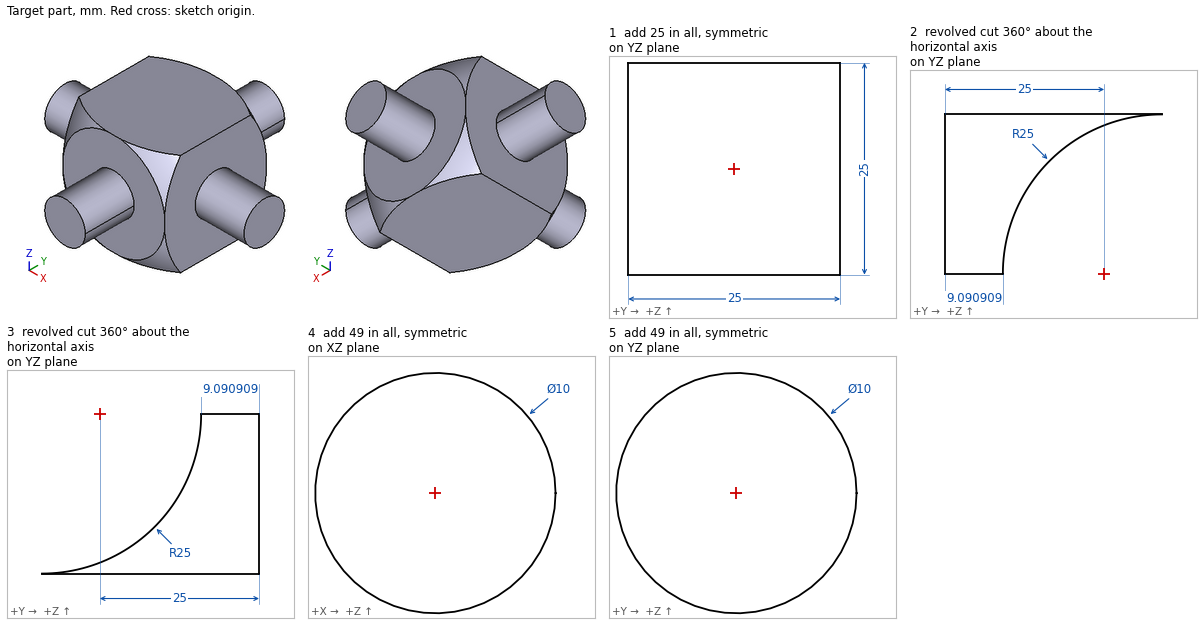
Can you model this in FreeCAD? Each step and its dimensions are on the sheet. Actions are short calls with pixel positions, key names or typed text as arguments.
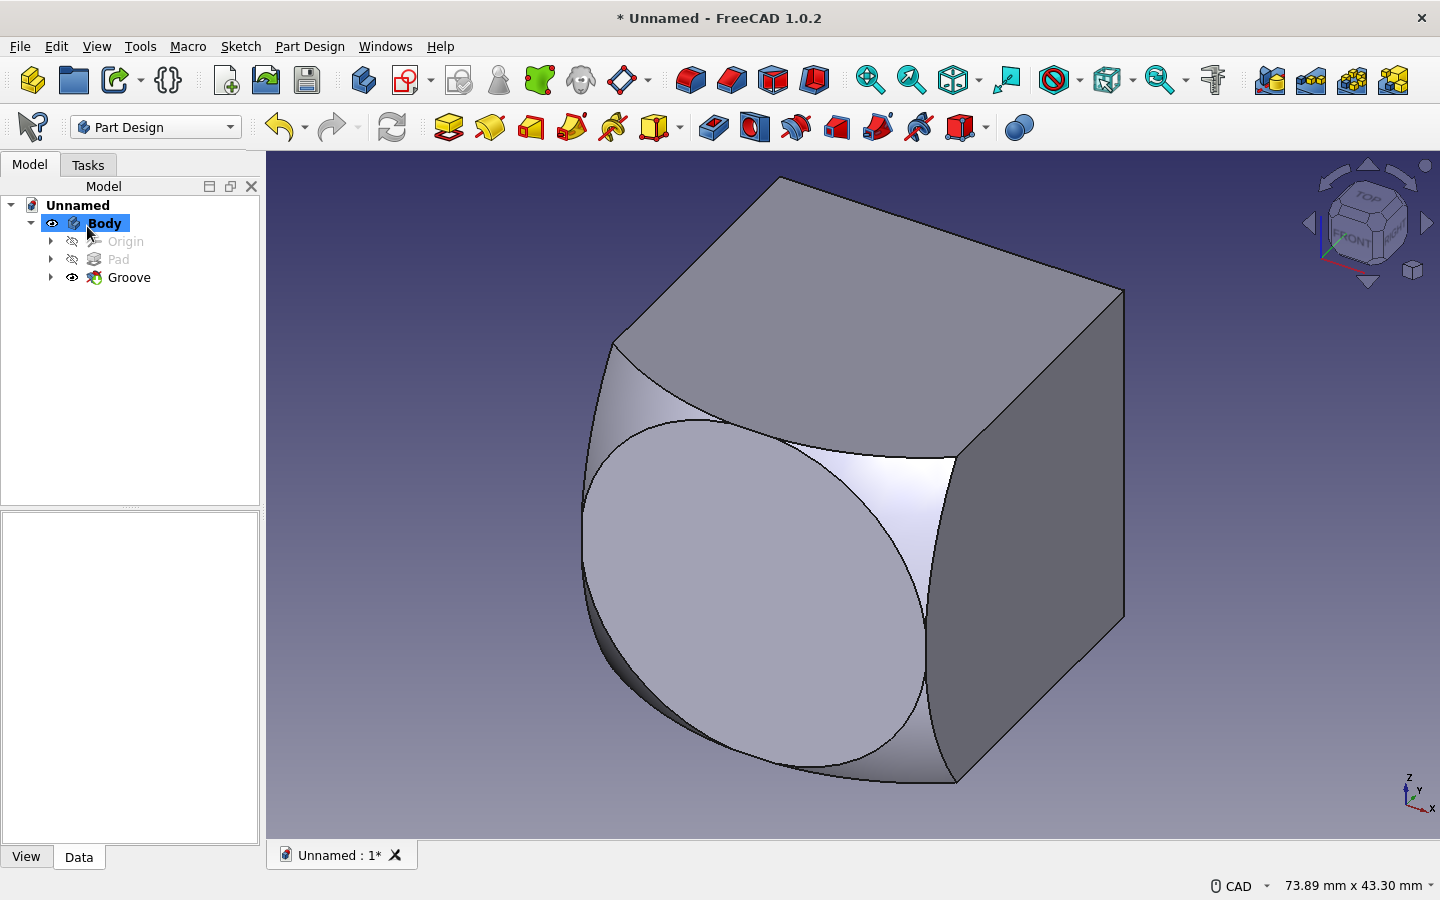
click(404, 80)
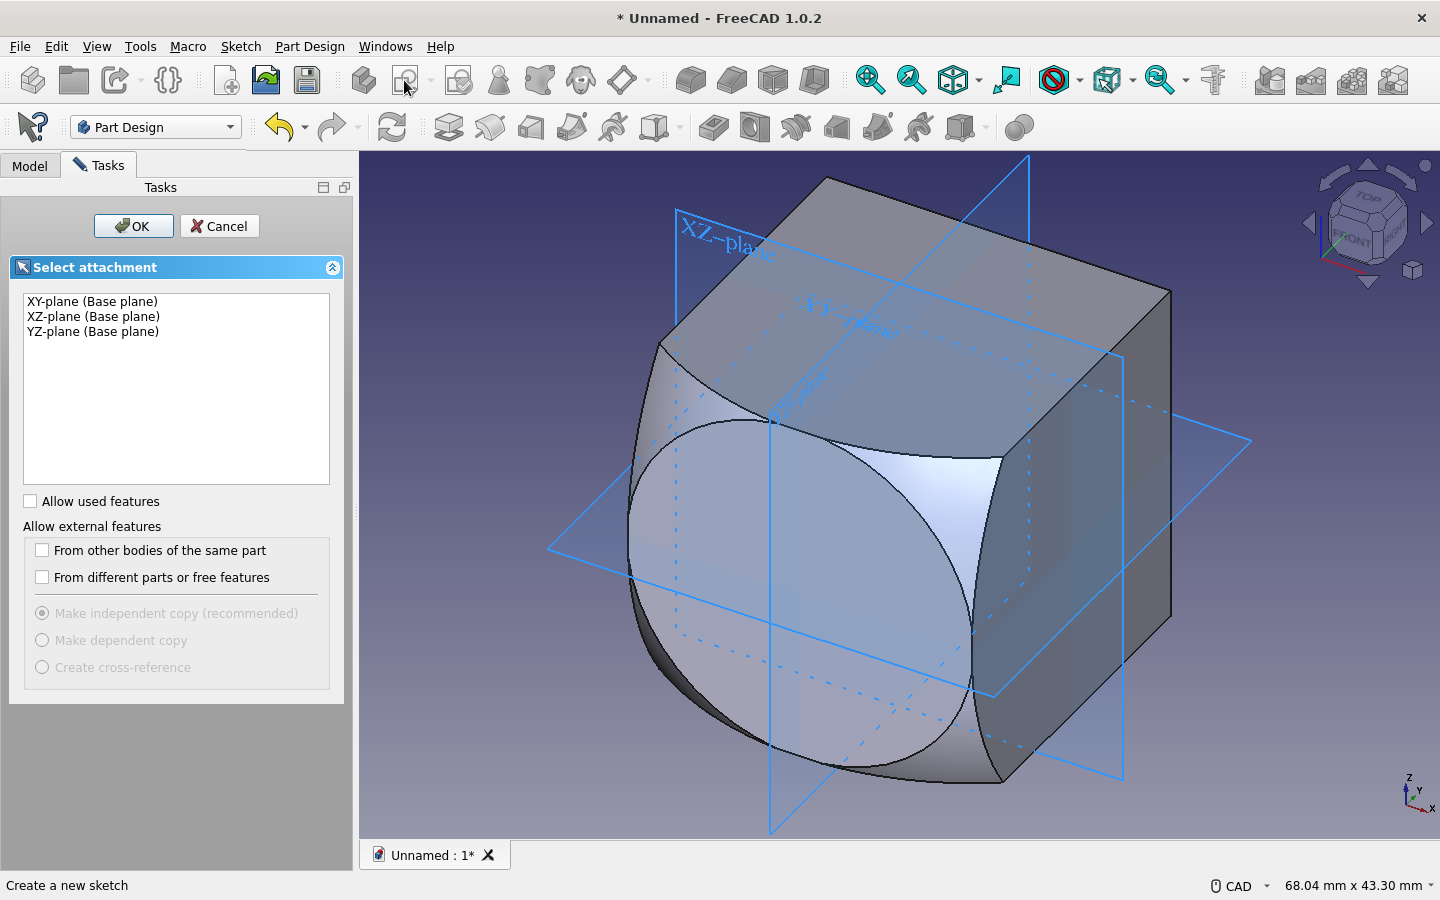
click(84, 332)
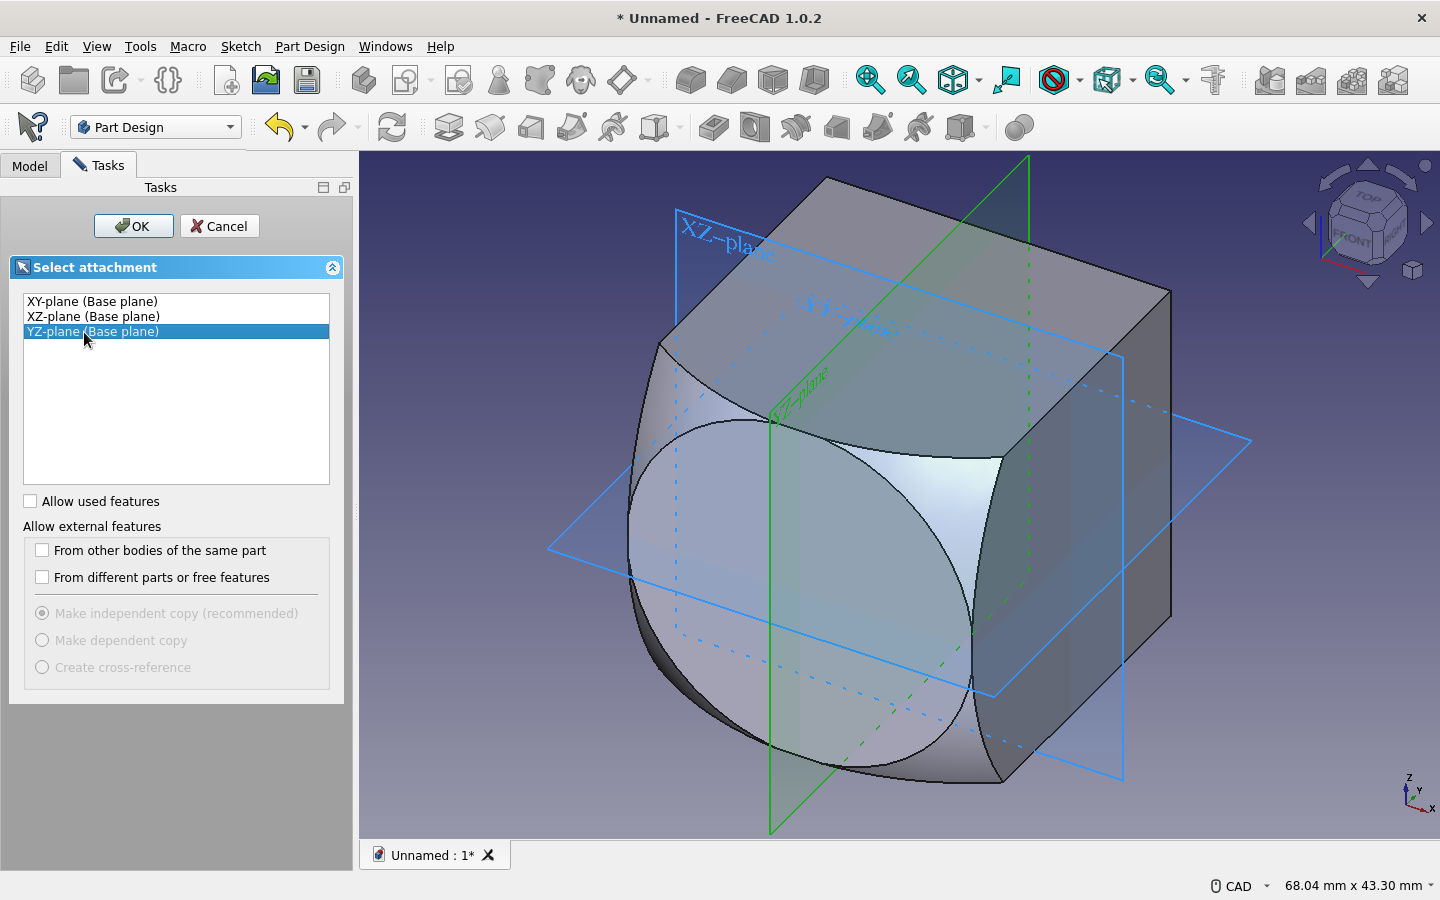
click(134, 226)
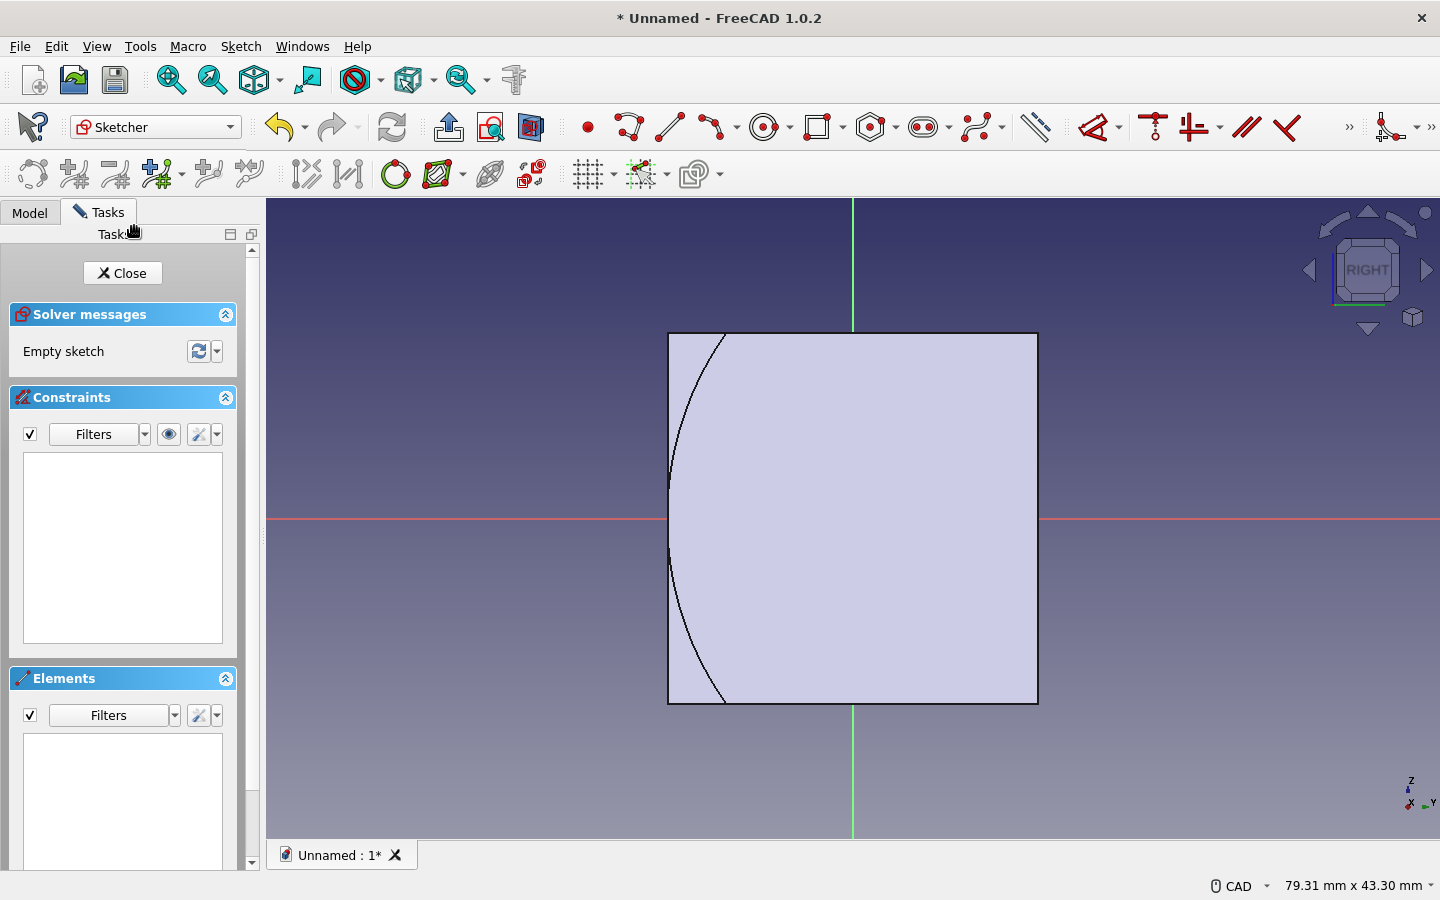
key(q)
key(s)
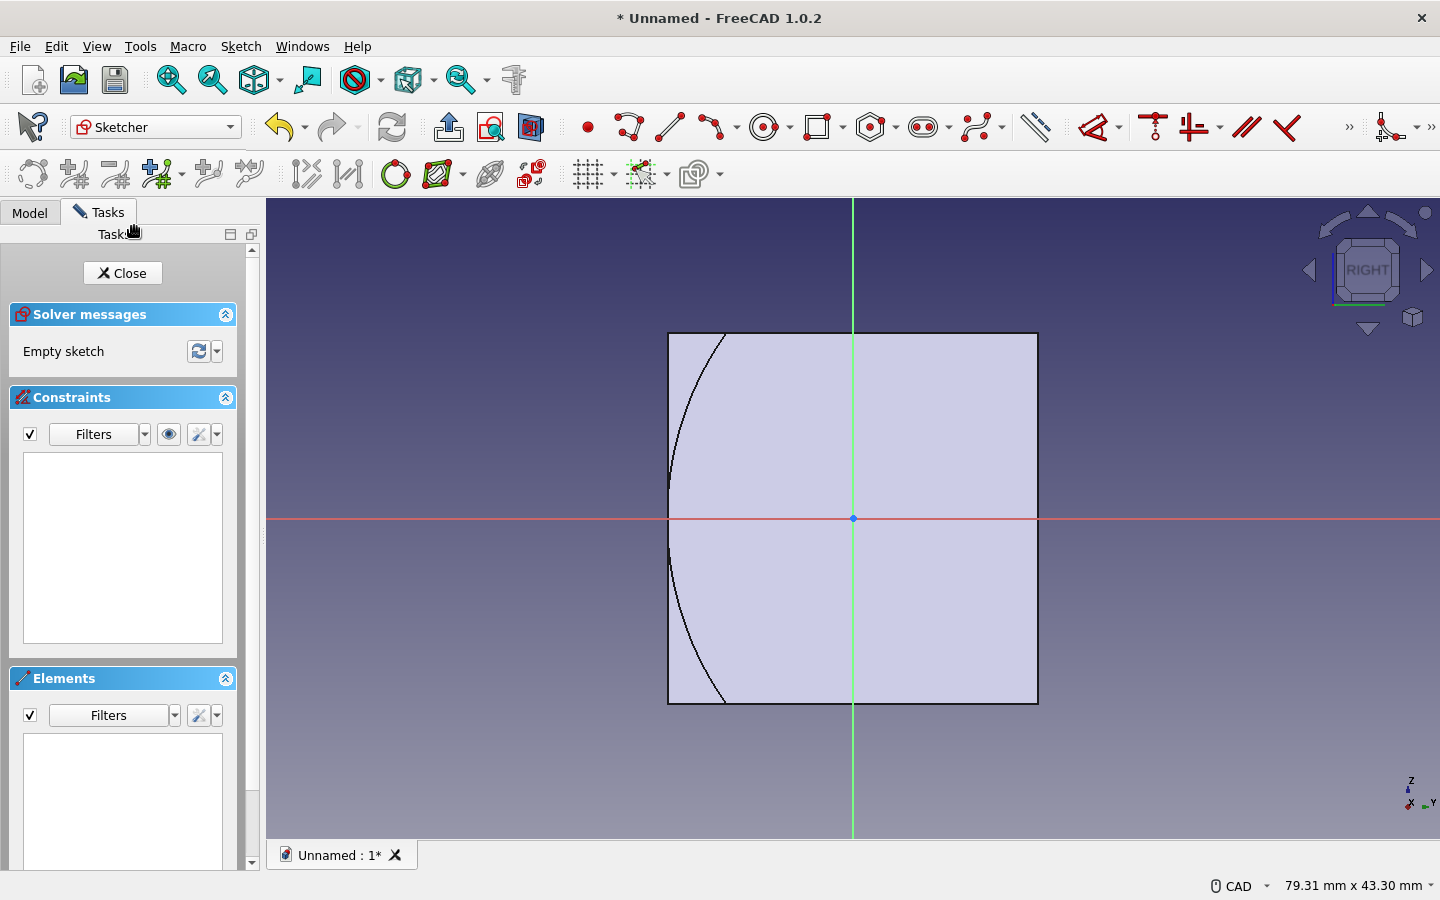
scroll(294, 226, down, 1)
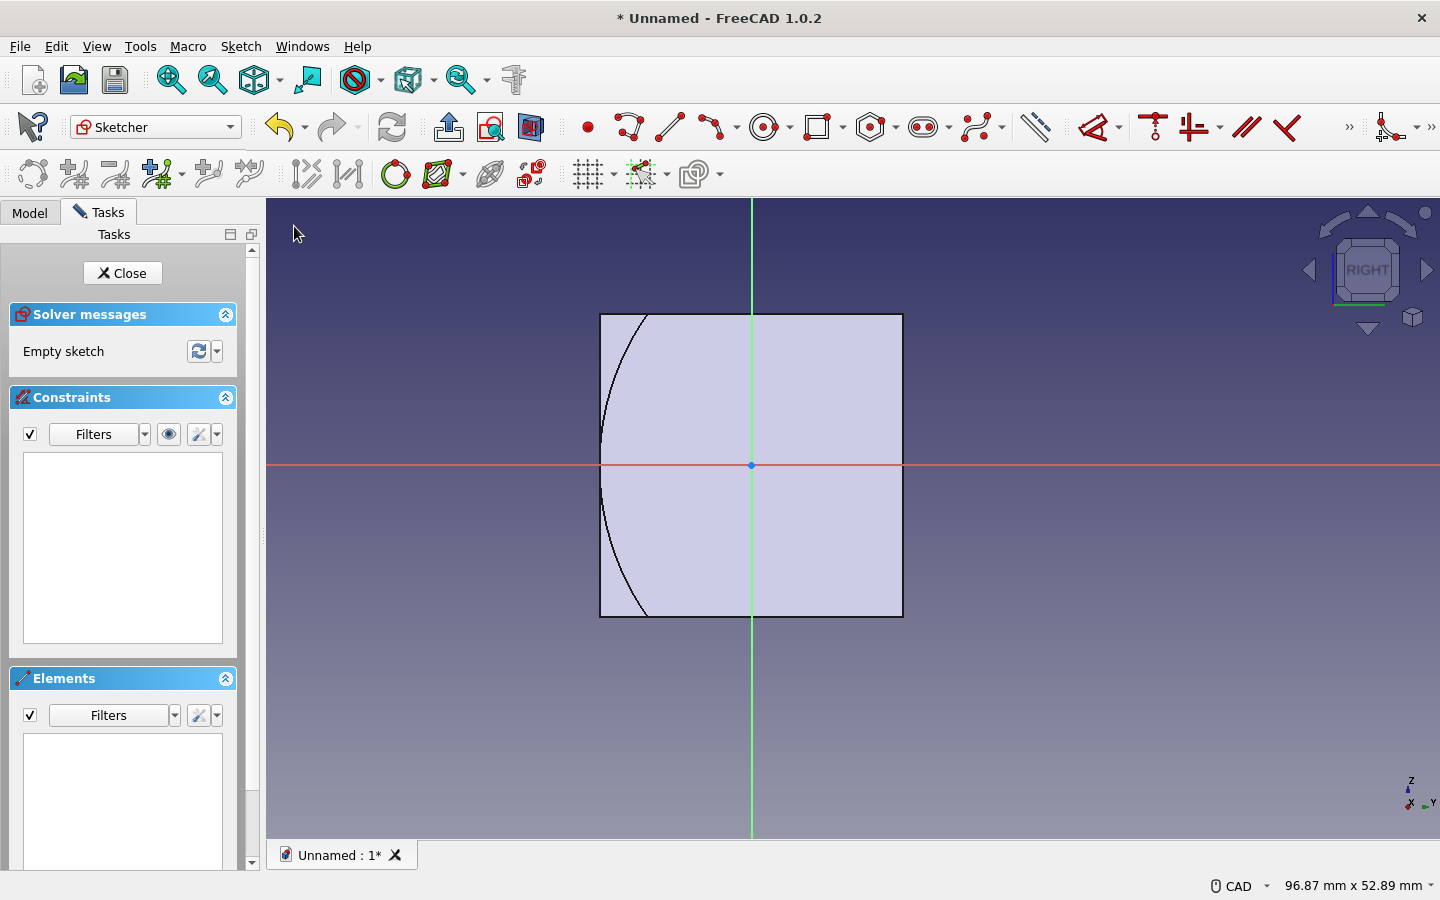
scroll(977, 811, up, 2)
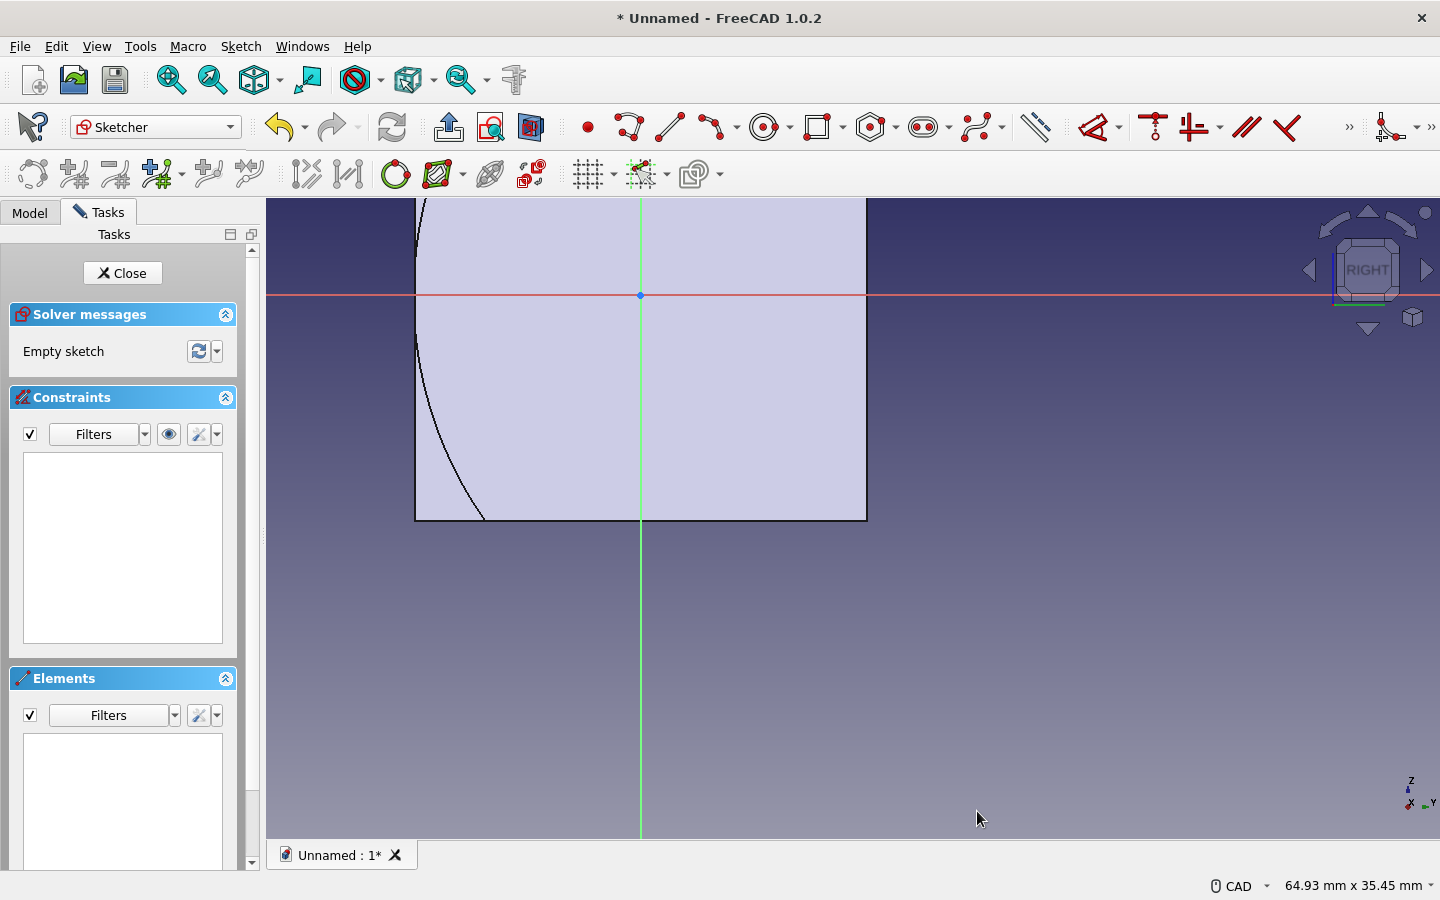
click(629, 128)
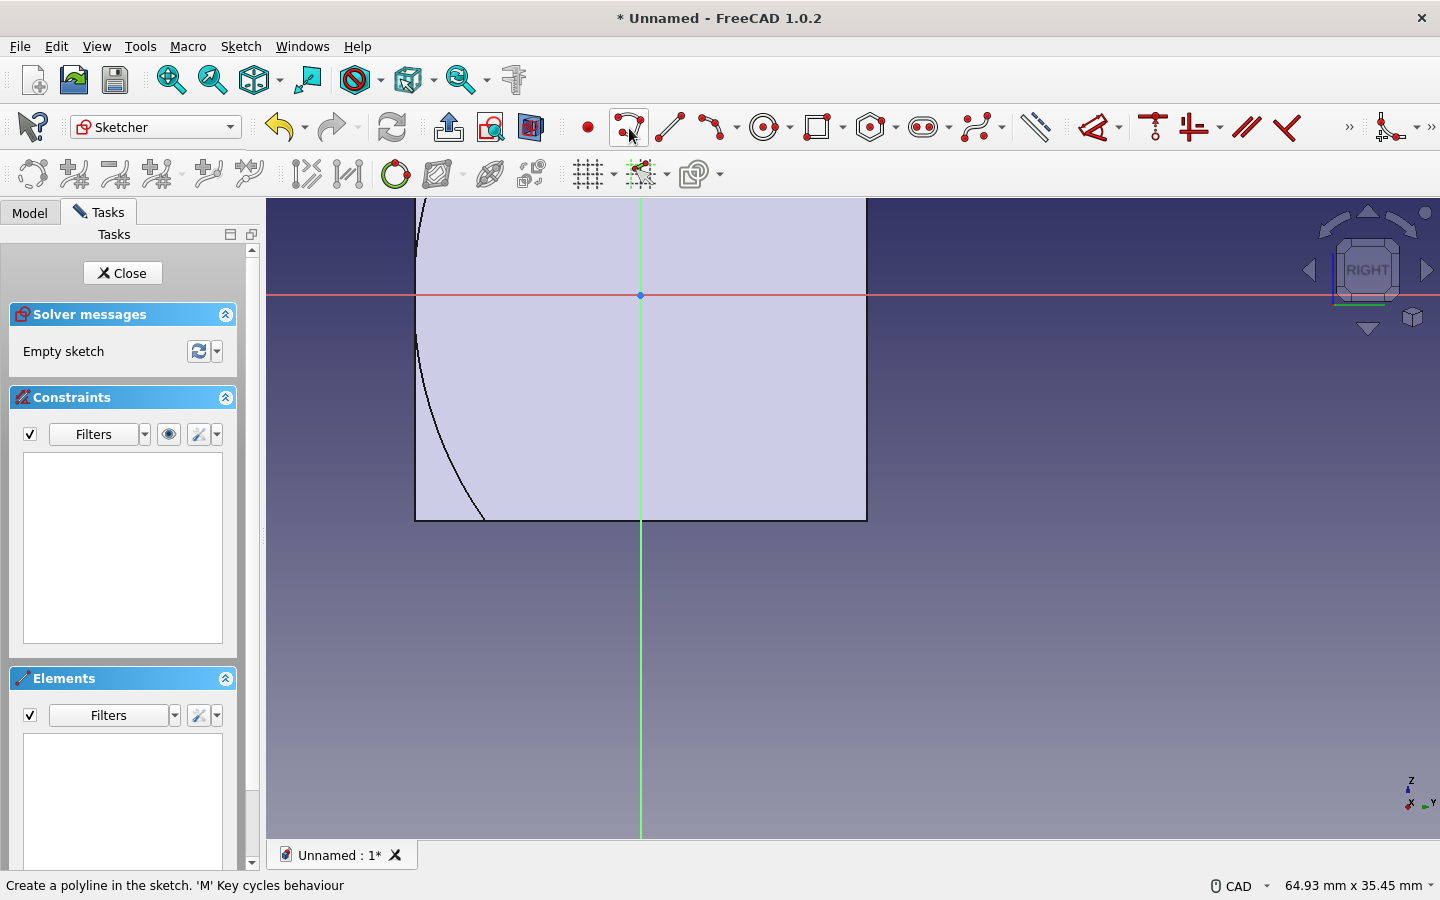
click(476, 747)
click(1093, 747)
click(1093, 295)
click(928, 304)
right_click(928, 304)